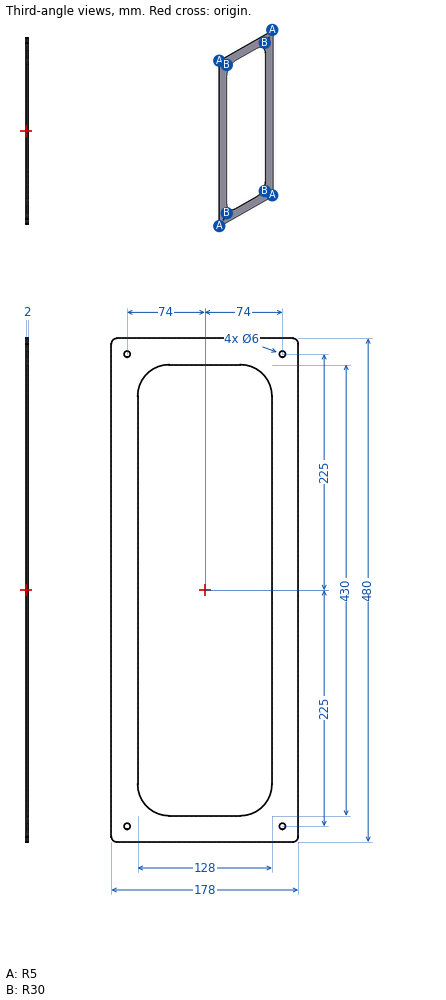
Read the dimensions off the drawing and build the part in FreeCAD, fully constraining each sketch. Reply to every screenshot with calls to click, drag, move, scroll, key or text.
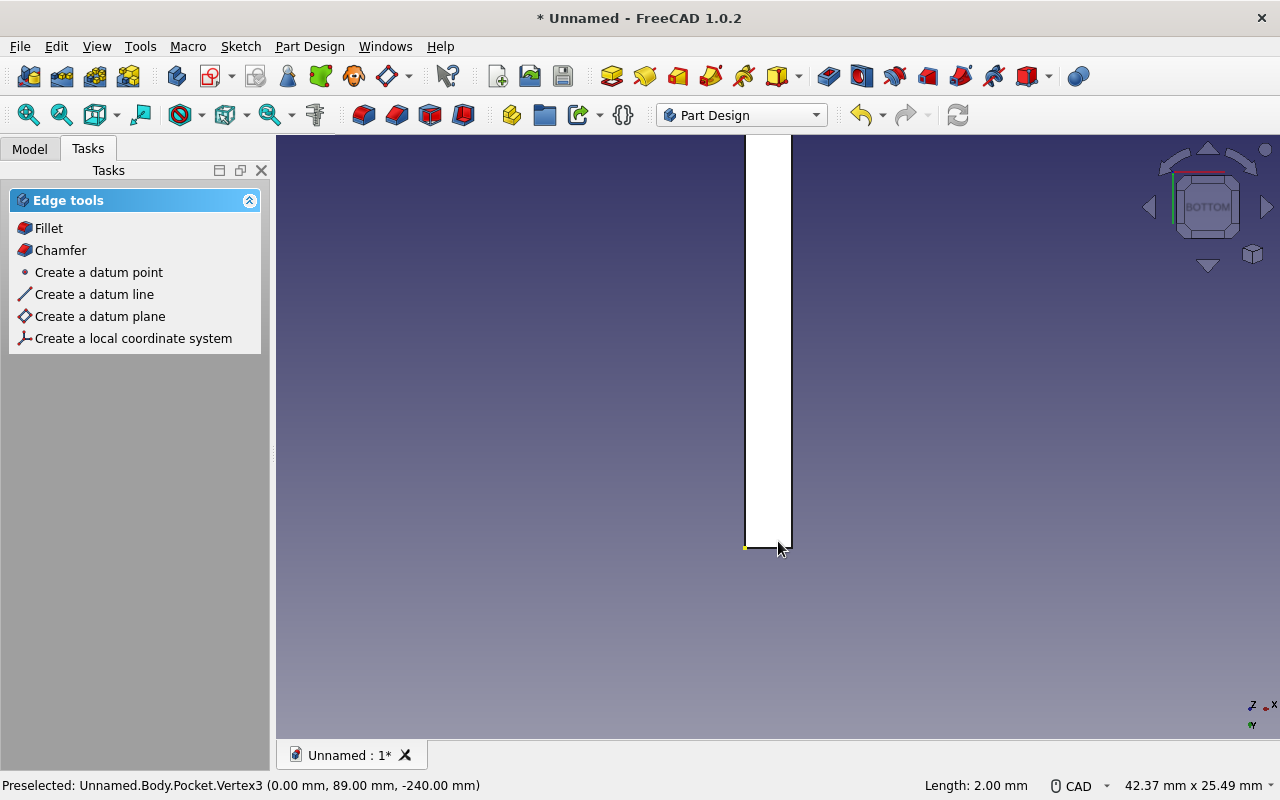
click(768, 547, ctrl)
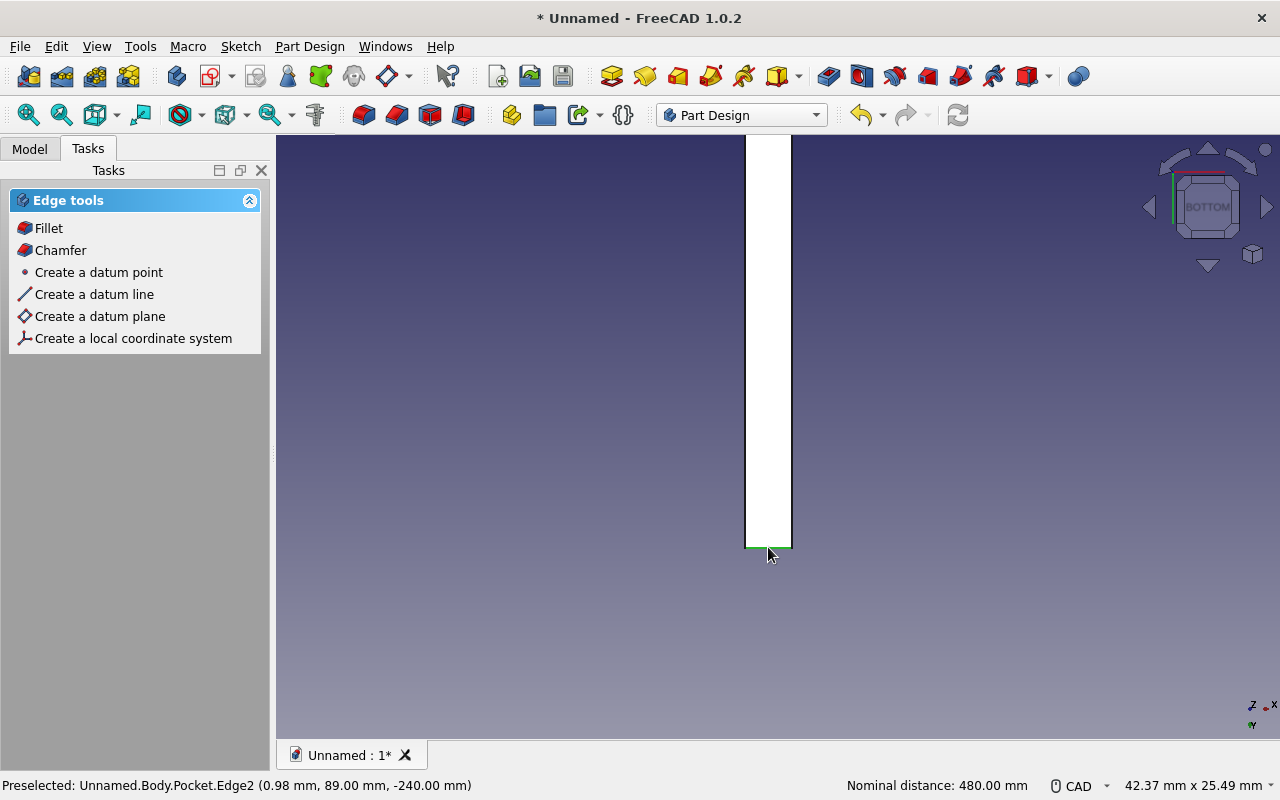
key(v)
key(f)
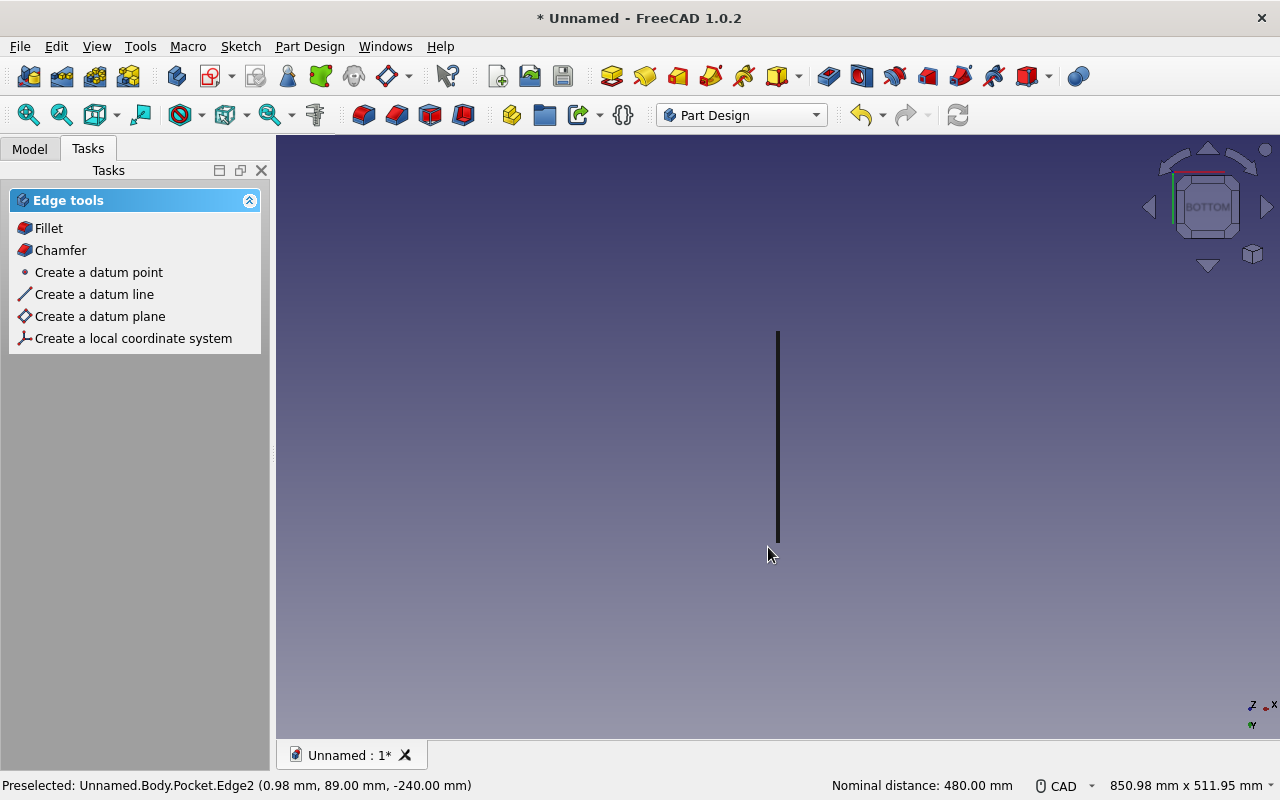
key(4)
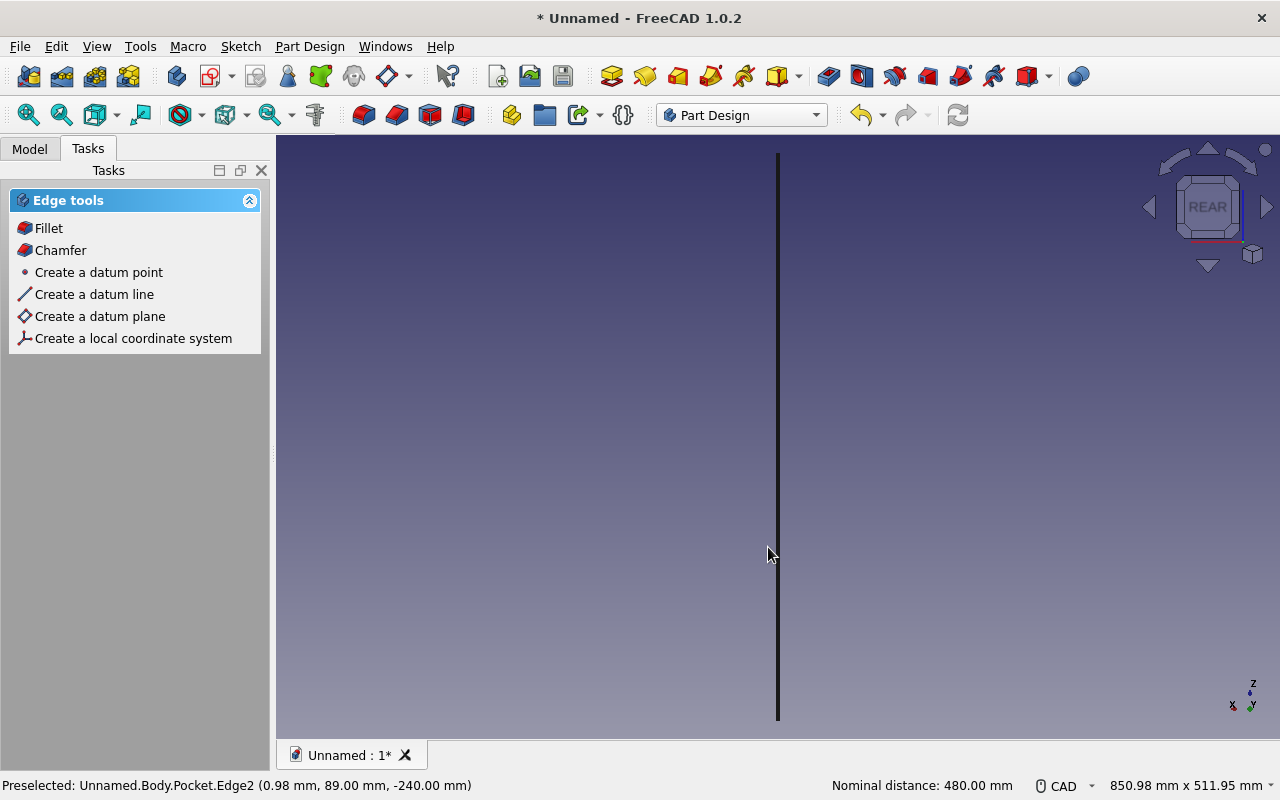
key(6)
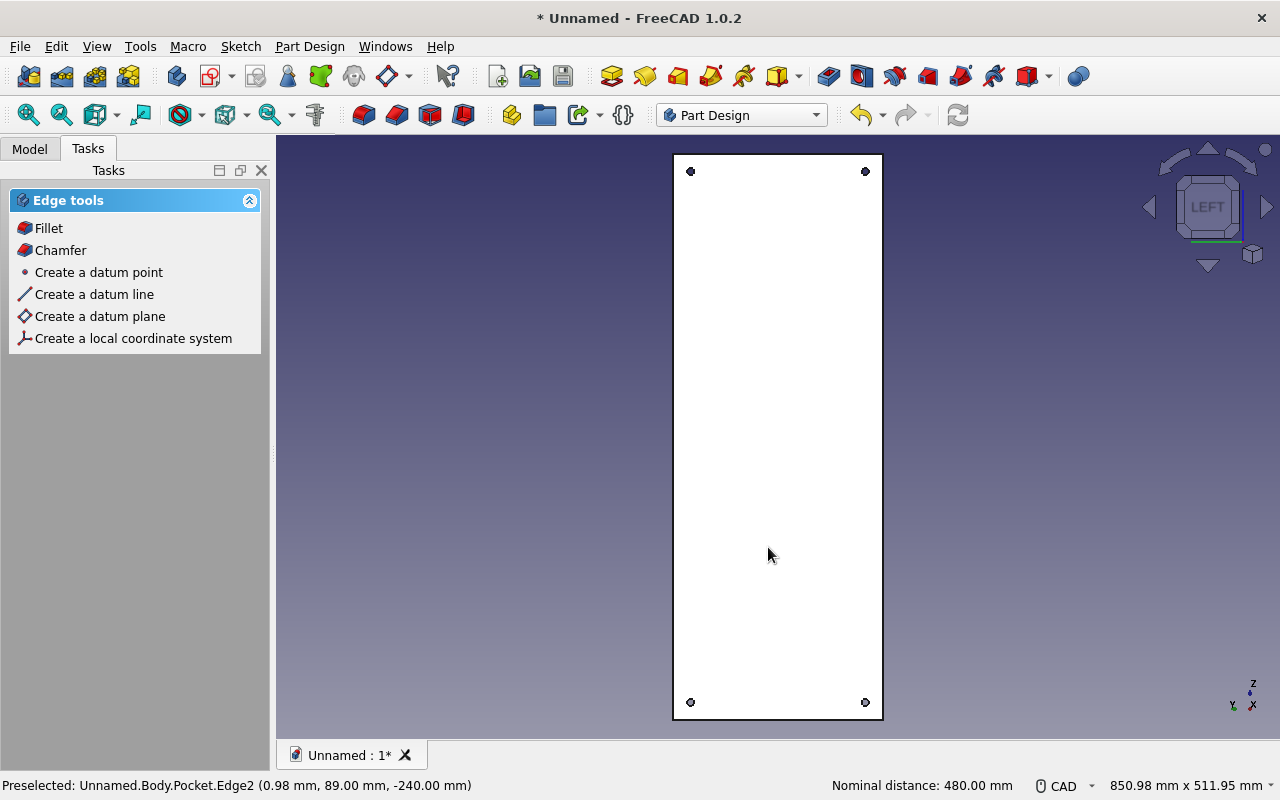
key(v)
key(3)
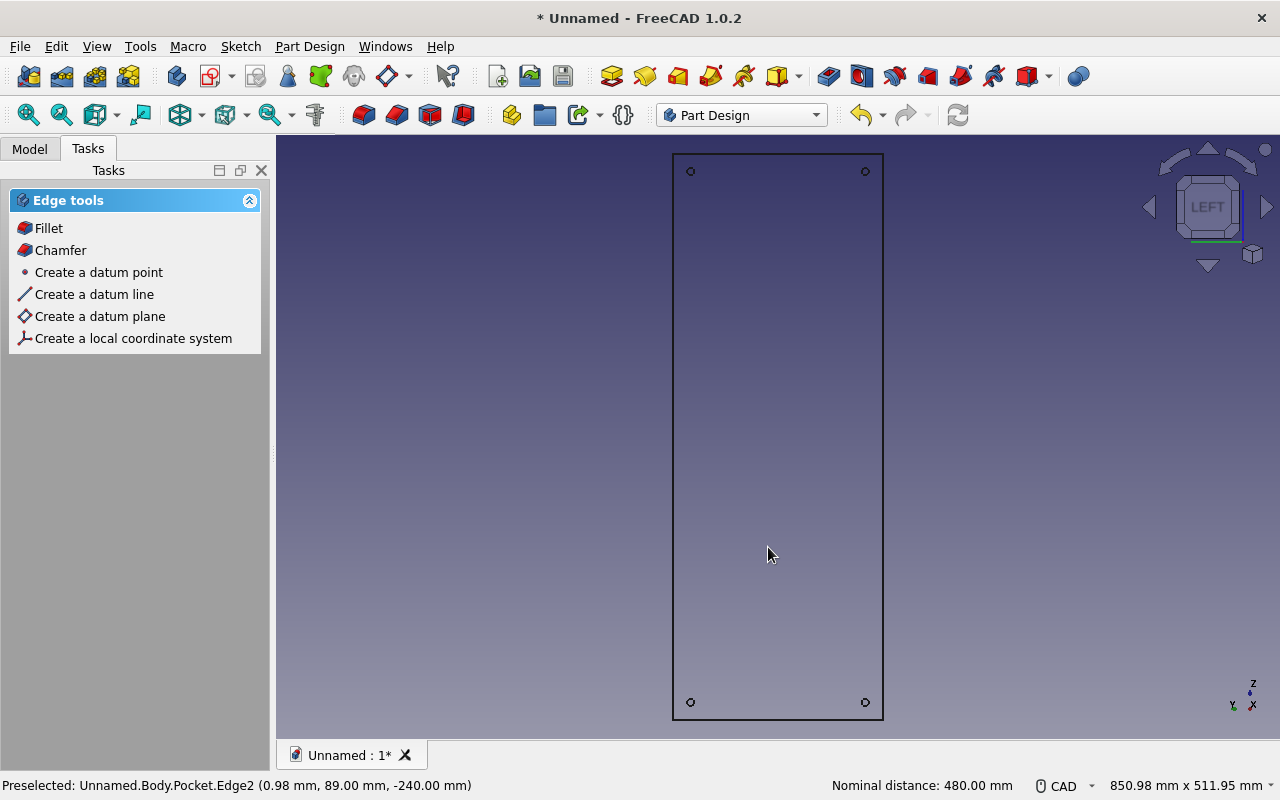
key(0)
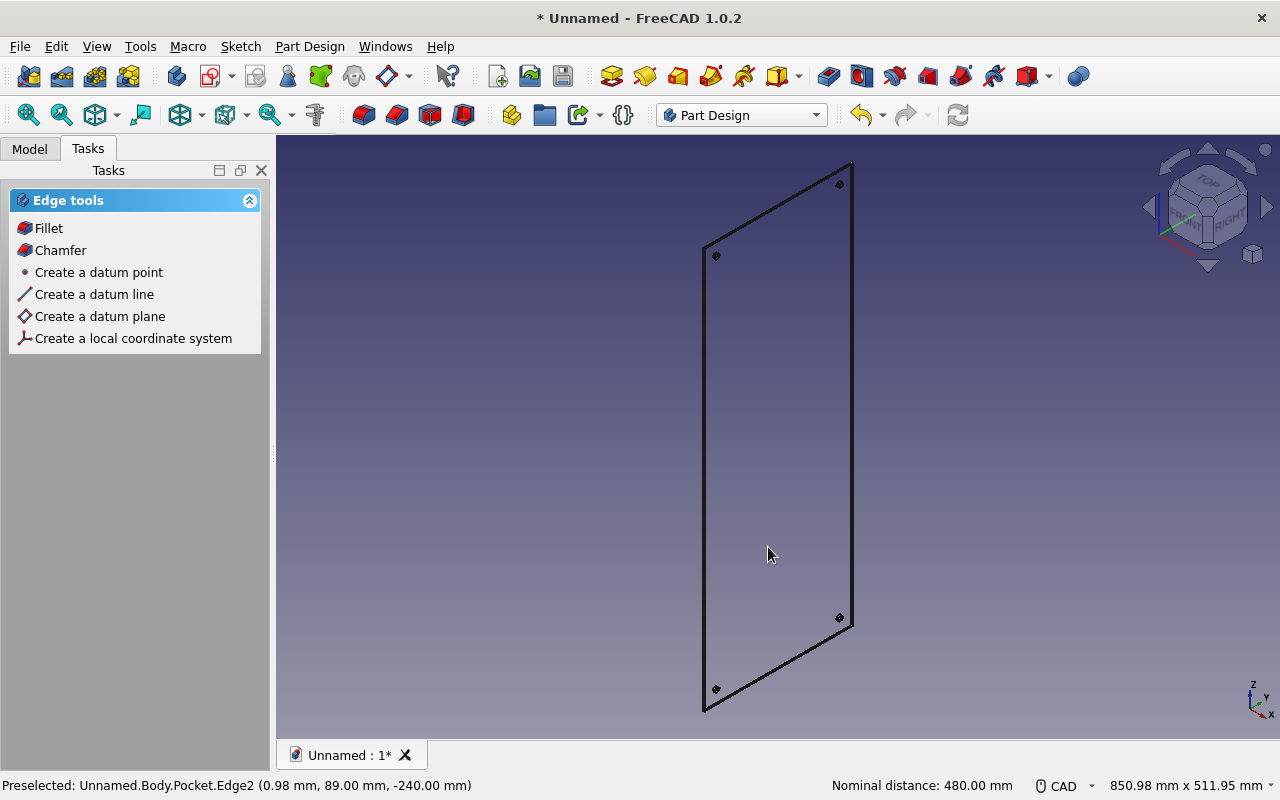
scroll(704, 710, up, 15)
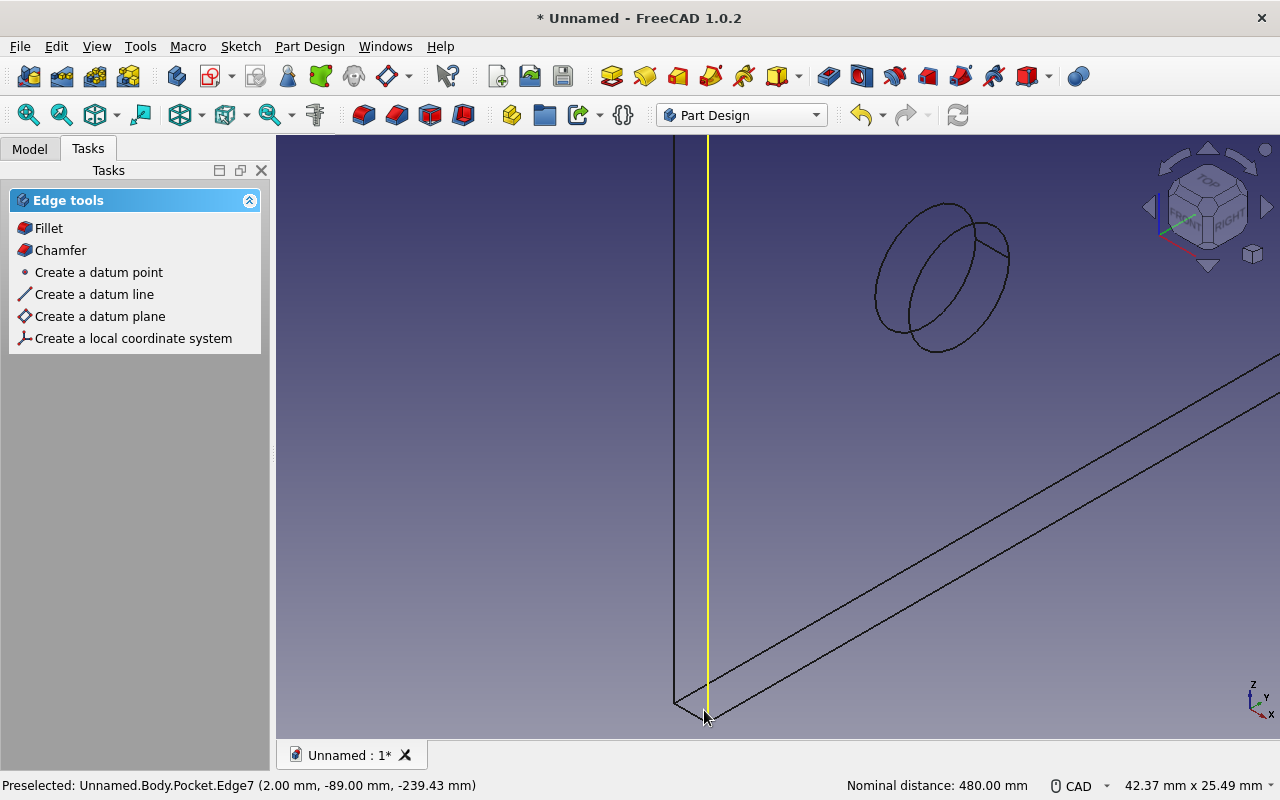
click(688, 710, ctrl)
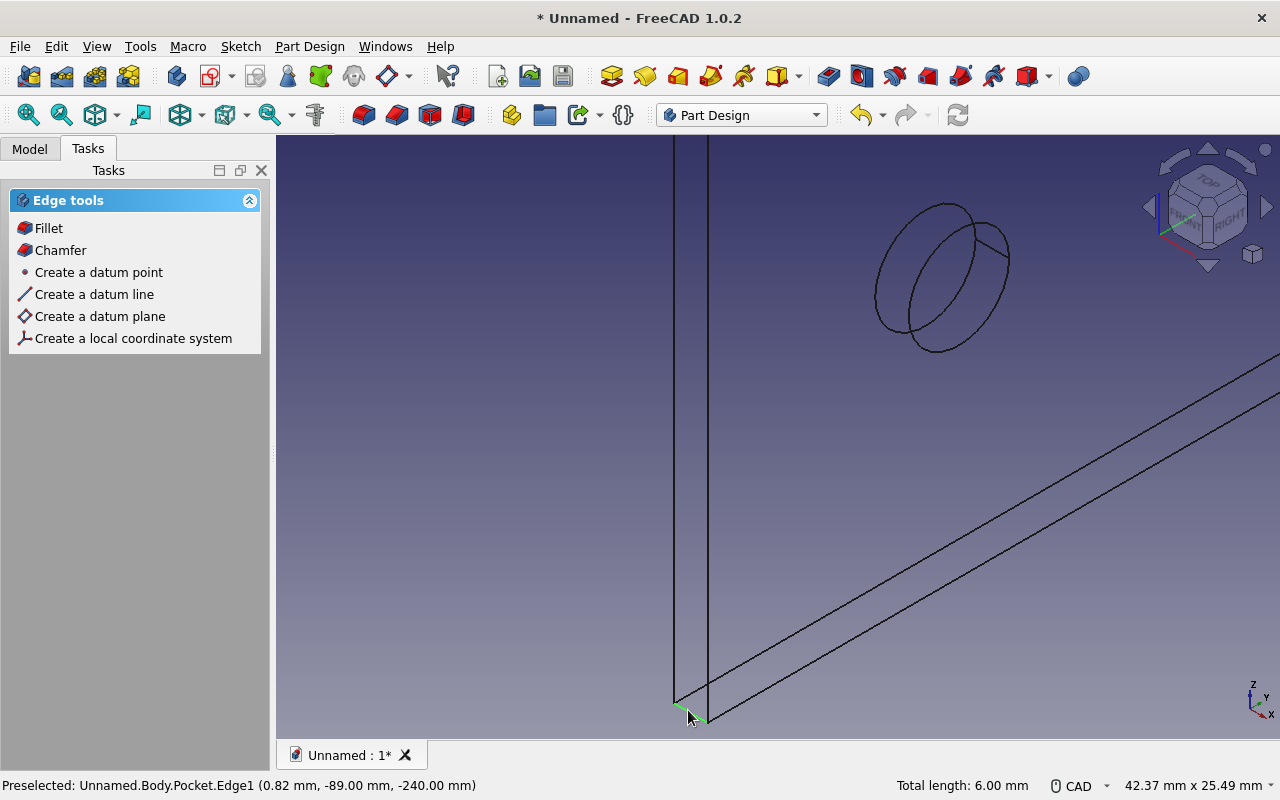
key(v)
key(f)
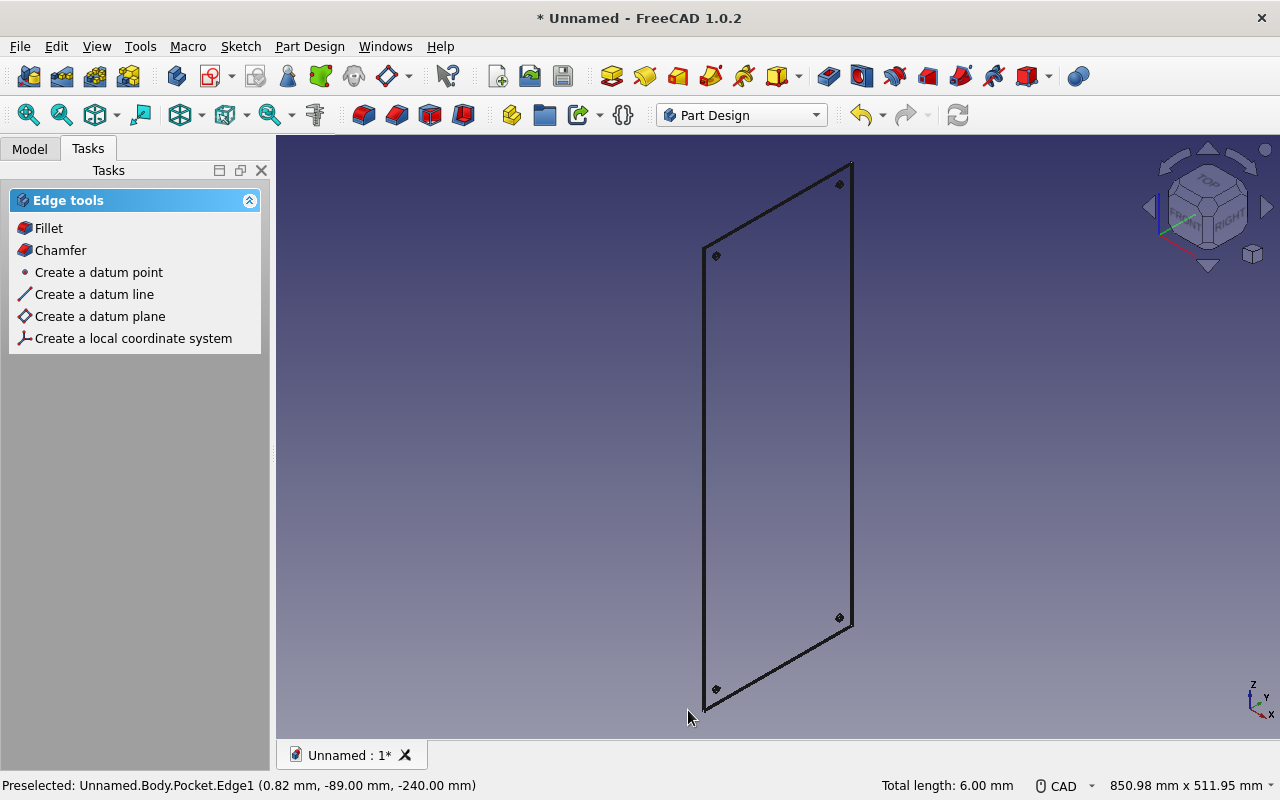
key(2)